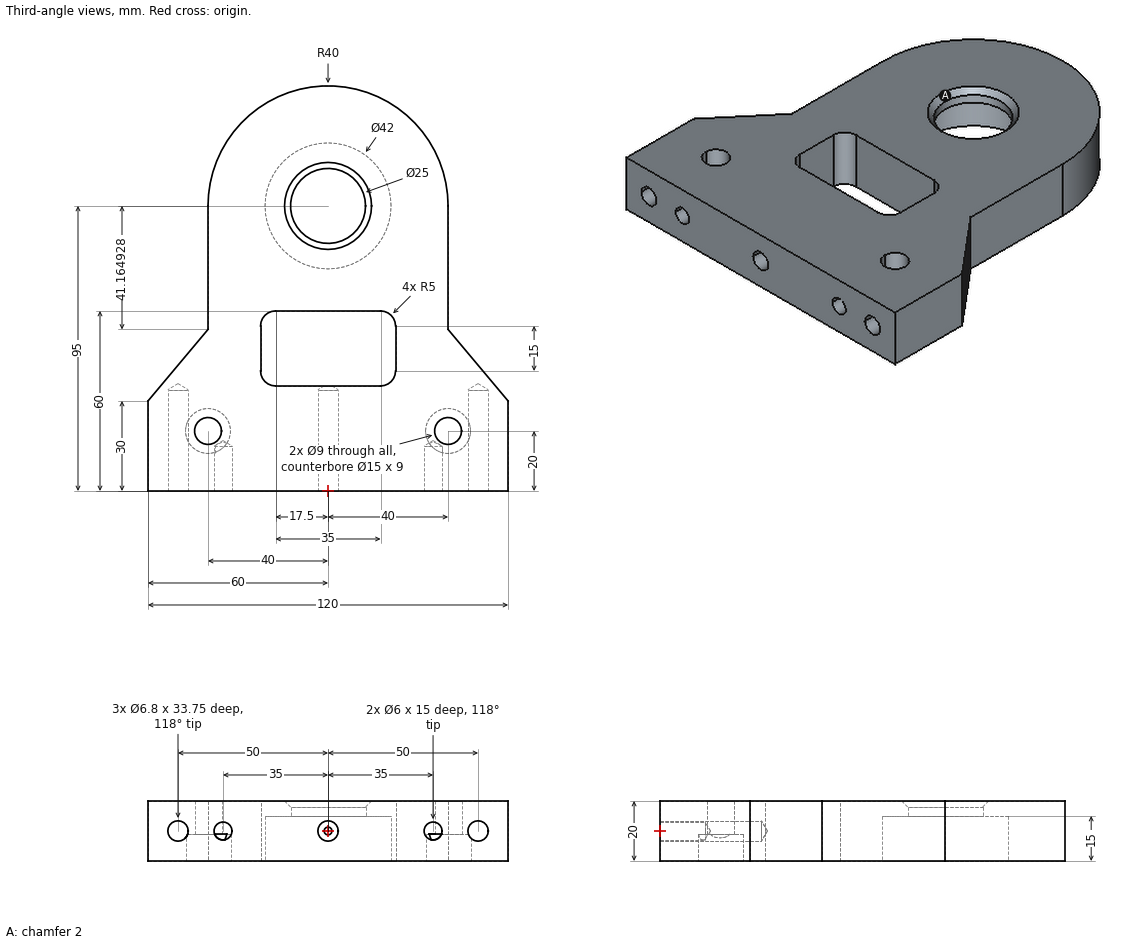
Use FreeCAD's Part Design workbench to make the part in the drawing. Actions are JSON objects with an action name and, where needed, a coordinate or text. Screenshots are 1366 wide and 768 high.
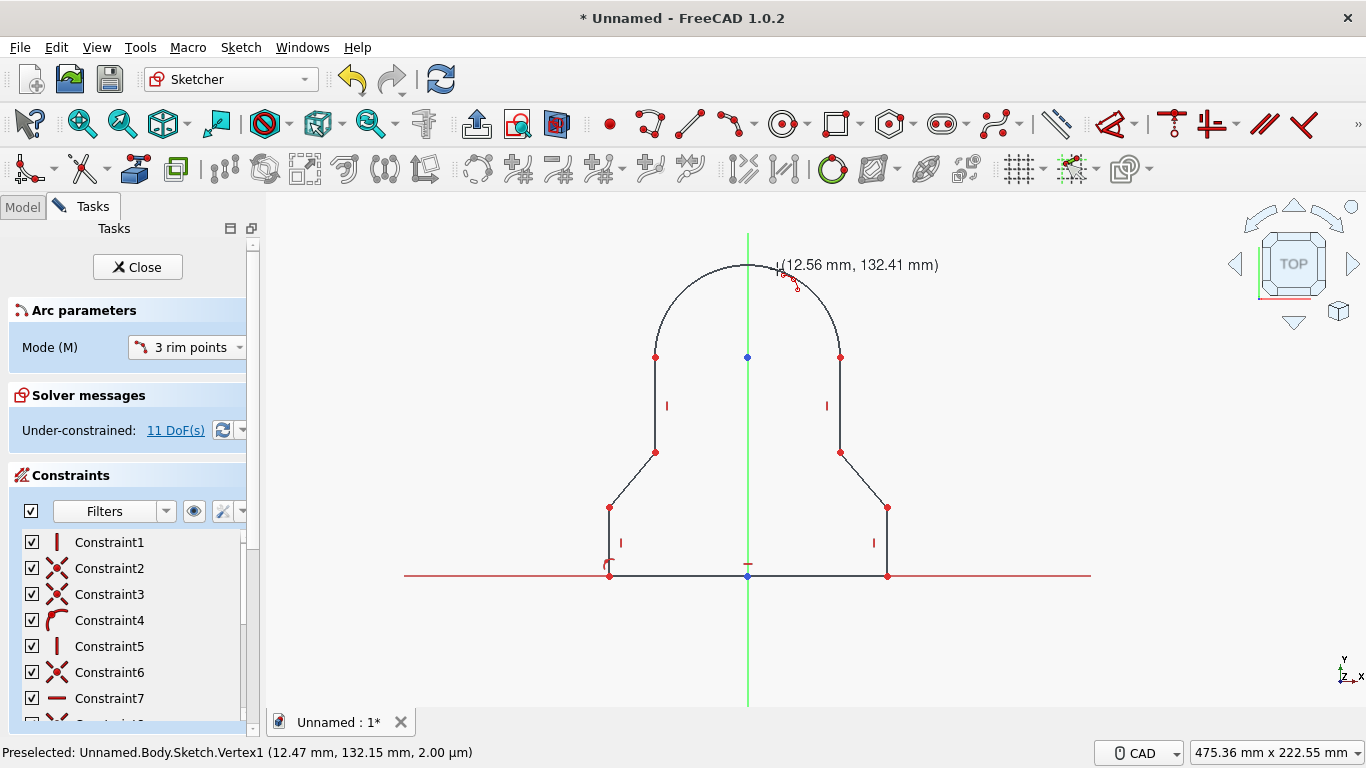
{"action": "left_click", "coordinate": [784, 124]}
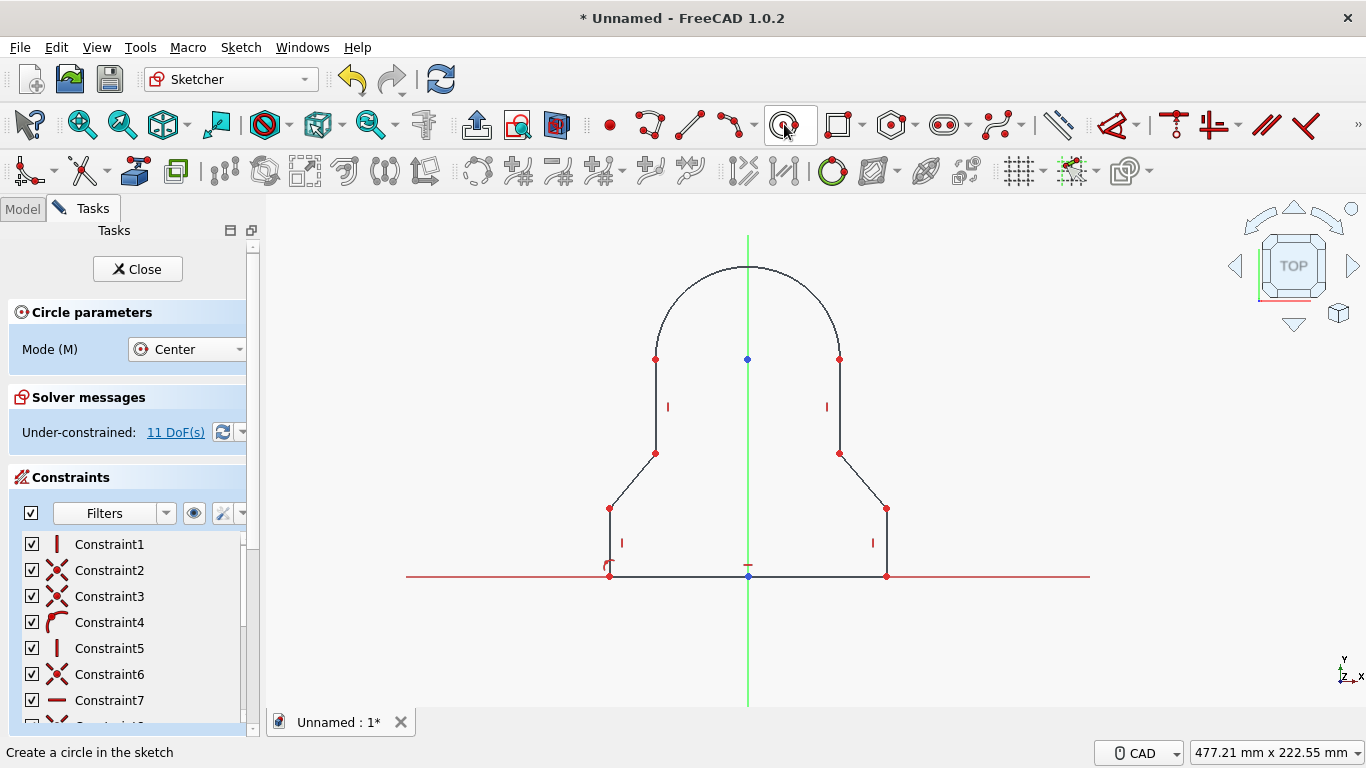
{"action": "left_click", "coordinate": [748, 358]}
{"action": "left_click", "coordinate": [769, 338]}
{"action": "key", "text": "Escape"}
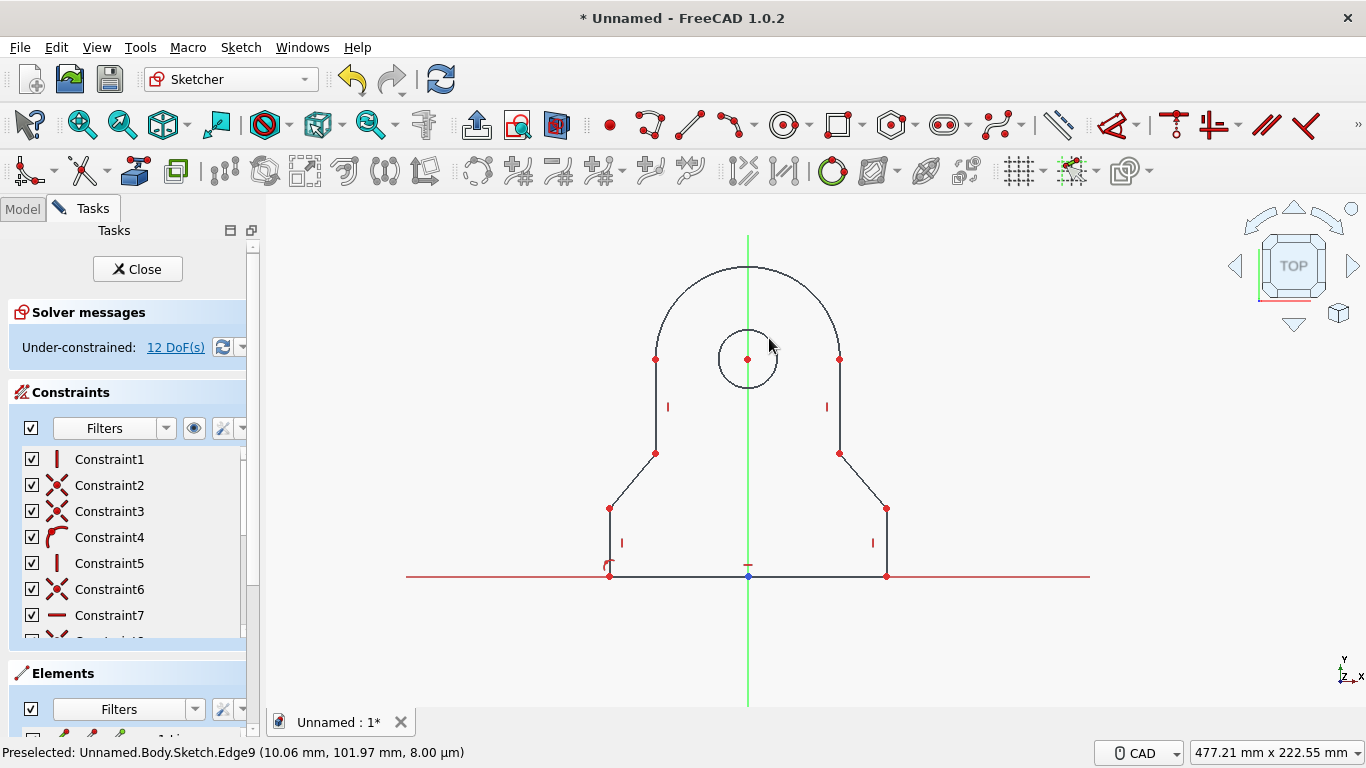
{"action": "left_click", "coordinate": [748, 359]}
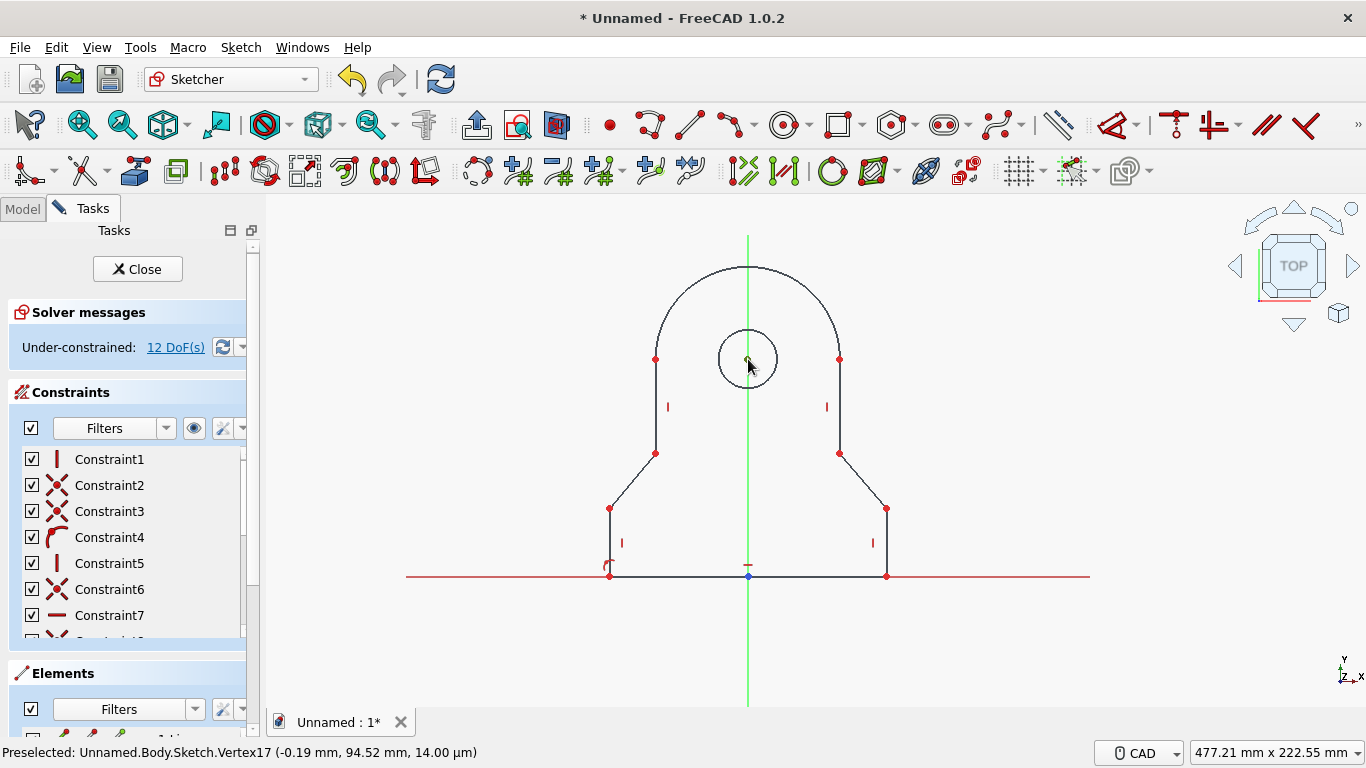
{"action": "left_click", "coordinate": [748, 646]}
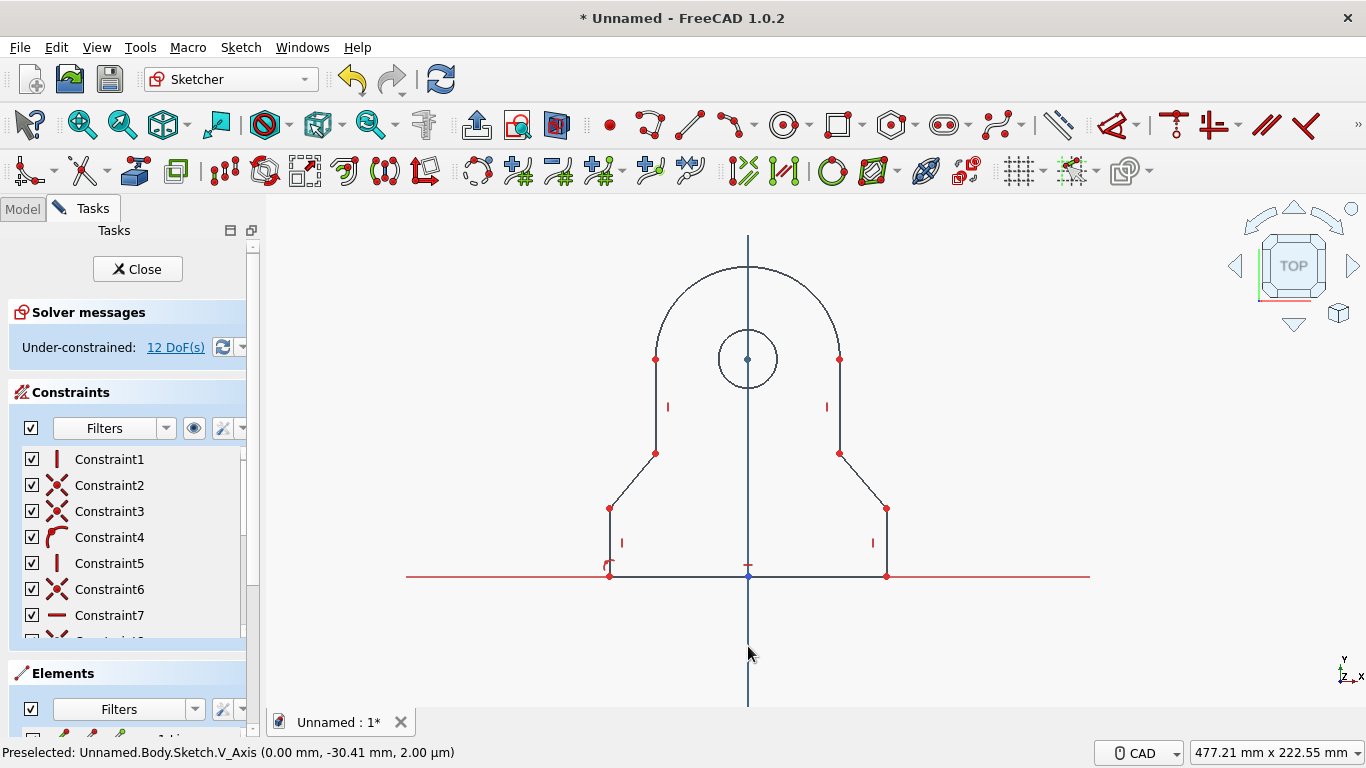
{"action": "left_click", "coordinate": [1174, 126]}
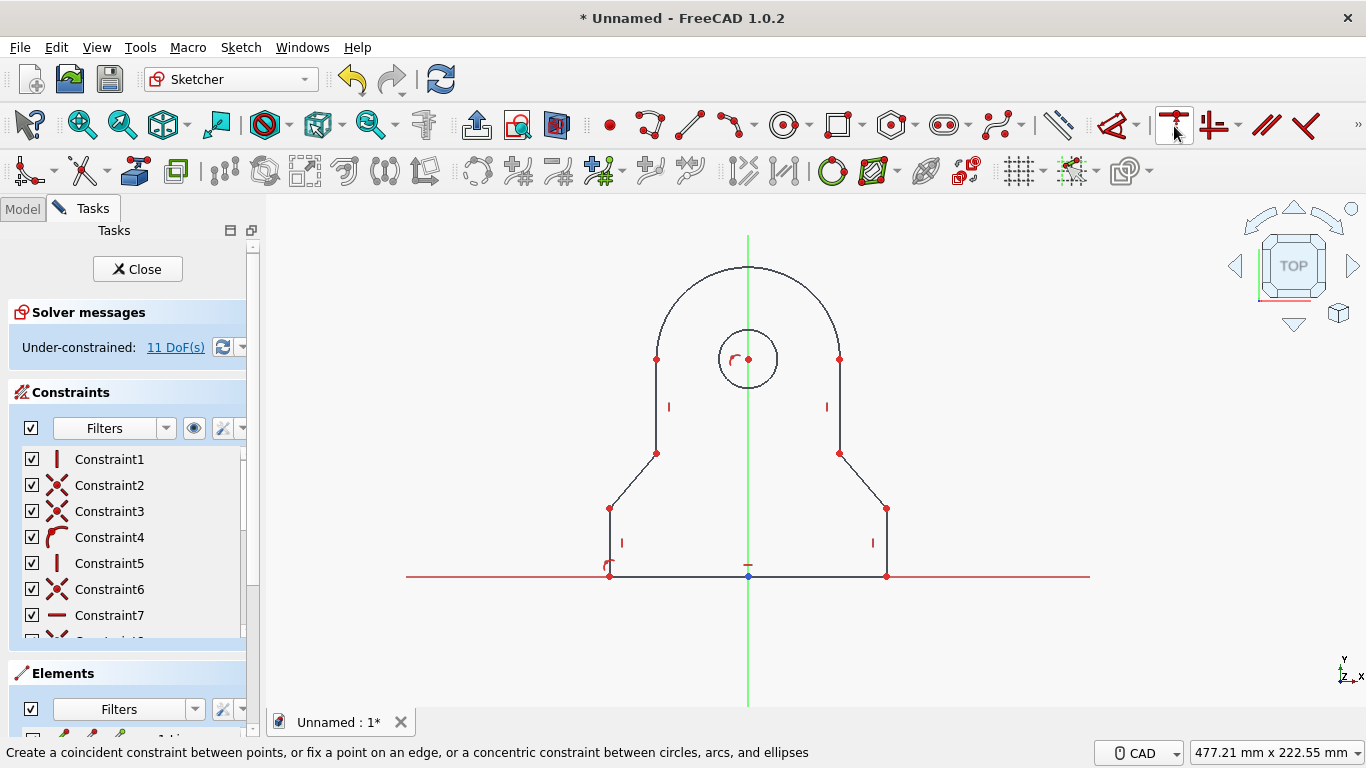
{"action": "left_click", "coordinate": [802, 285]}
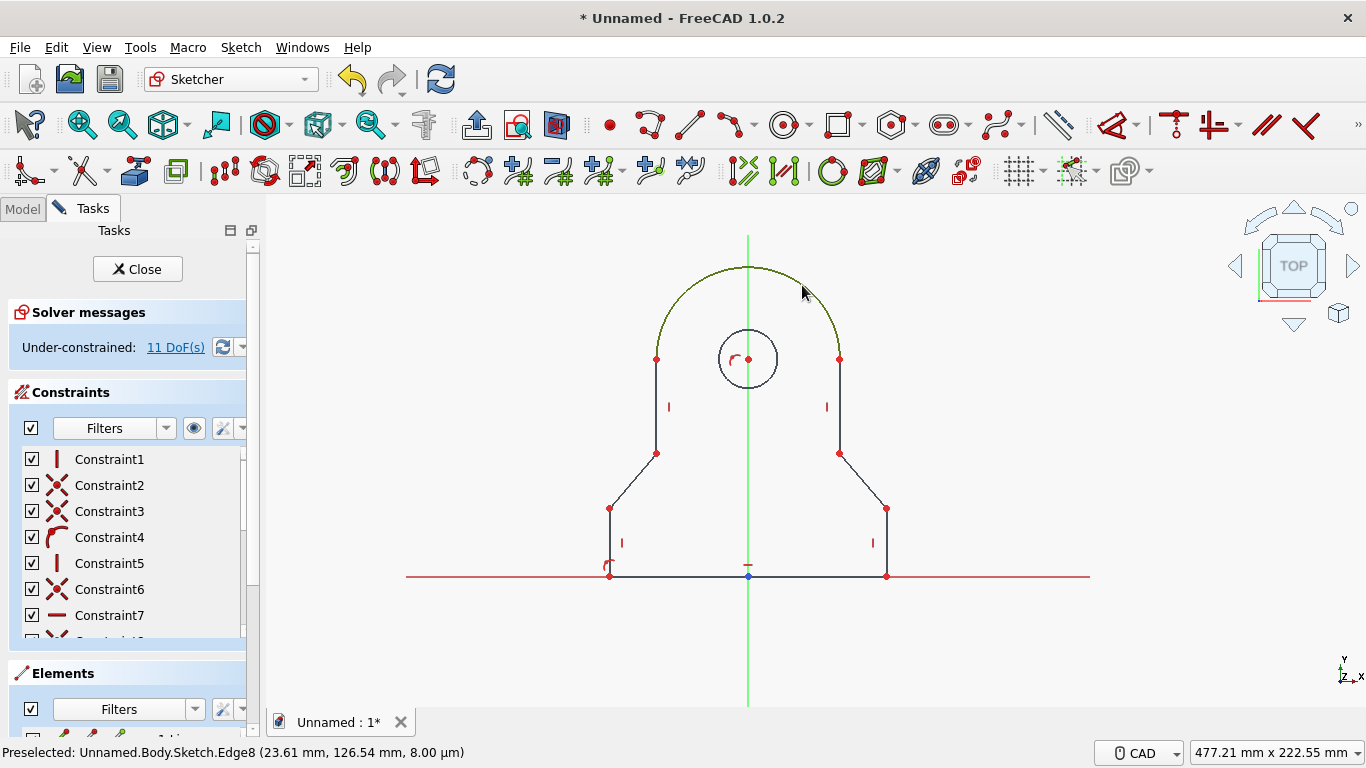
{"action": "key", "text": "k r"}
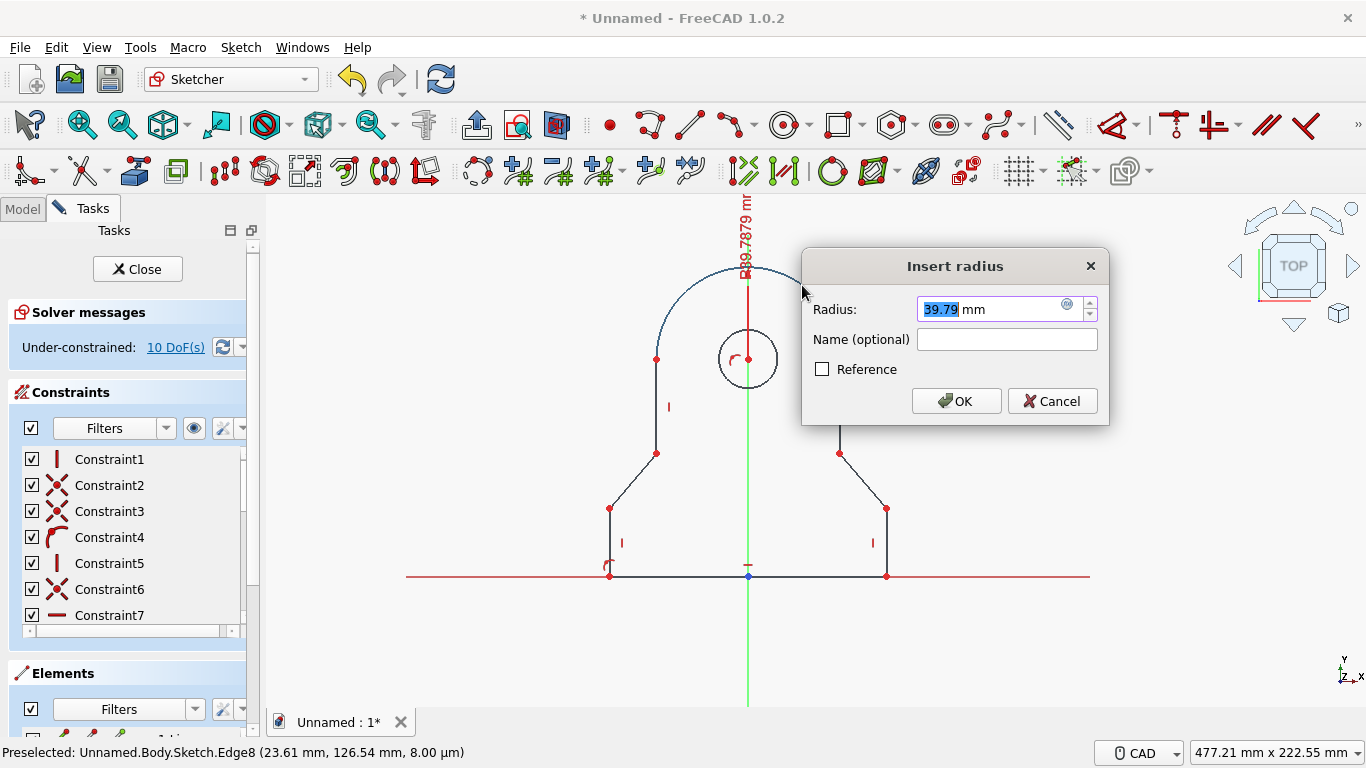
{"action": "type", "text": "40"}
{"action": "key", "text": "Return"}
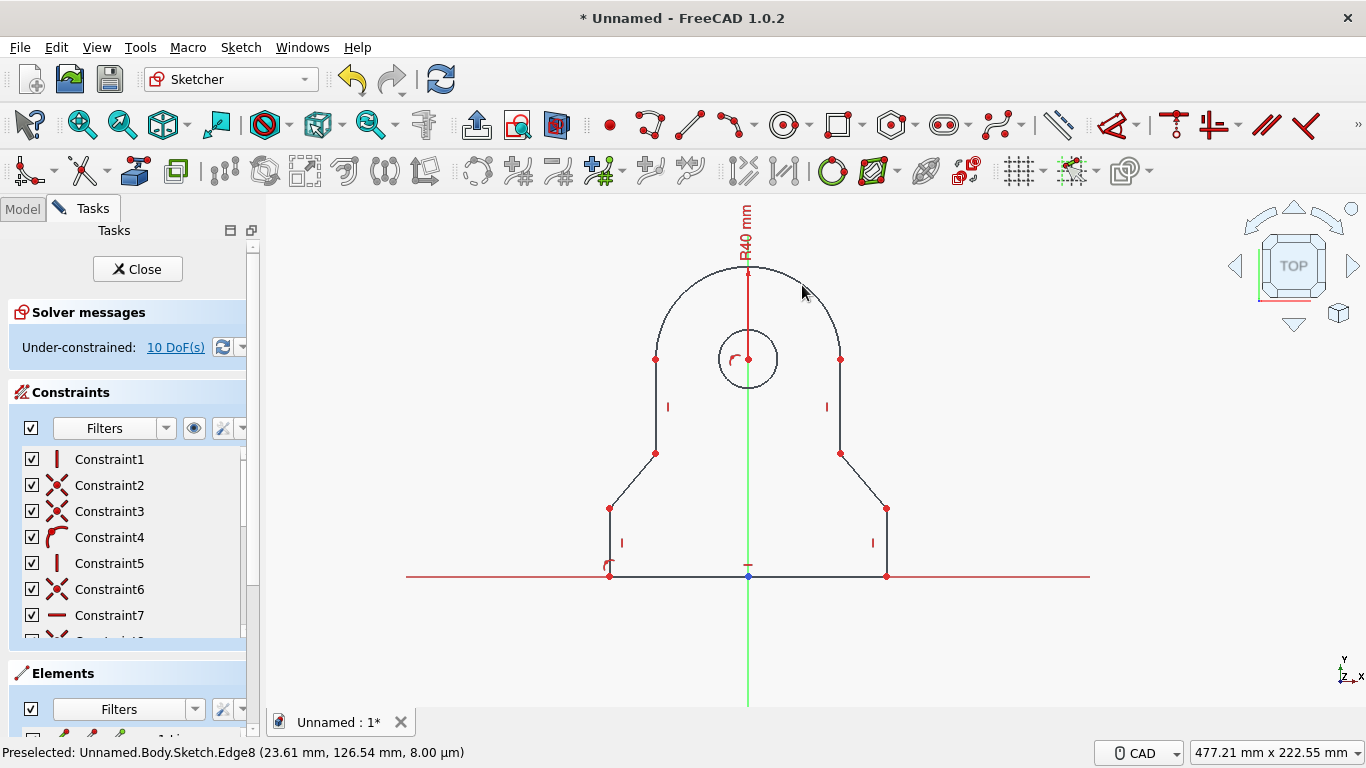
{"action": "left_click", "coordinate": [769, 338]}